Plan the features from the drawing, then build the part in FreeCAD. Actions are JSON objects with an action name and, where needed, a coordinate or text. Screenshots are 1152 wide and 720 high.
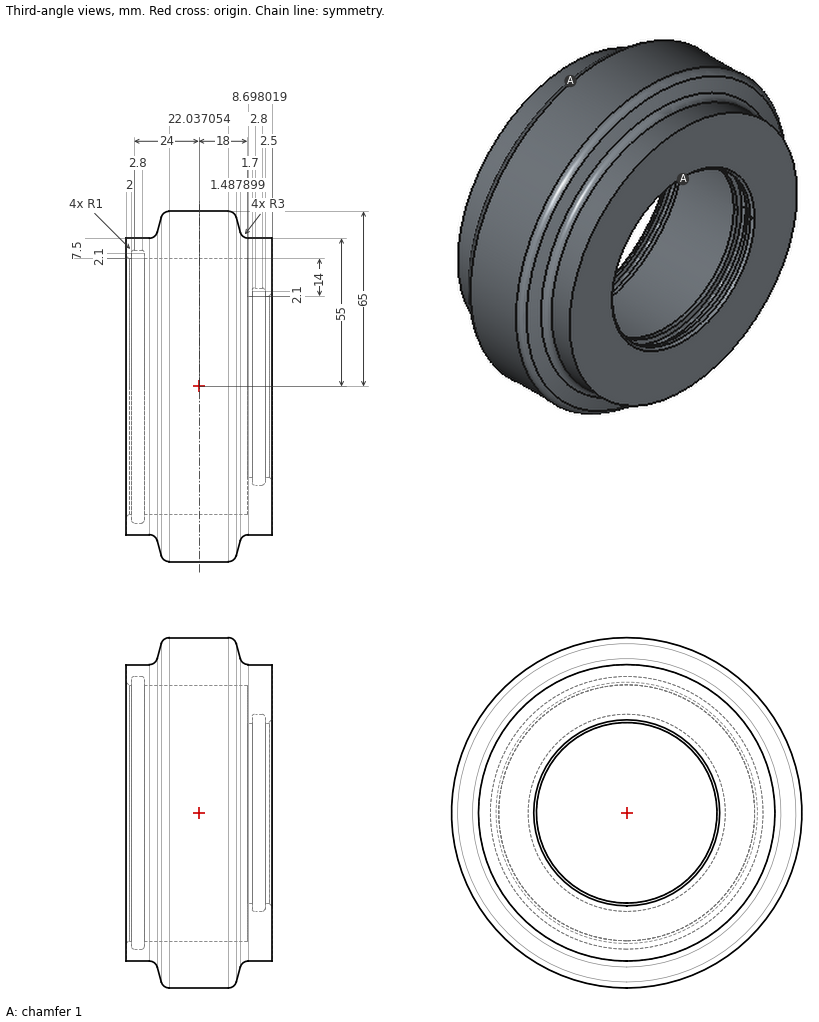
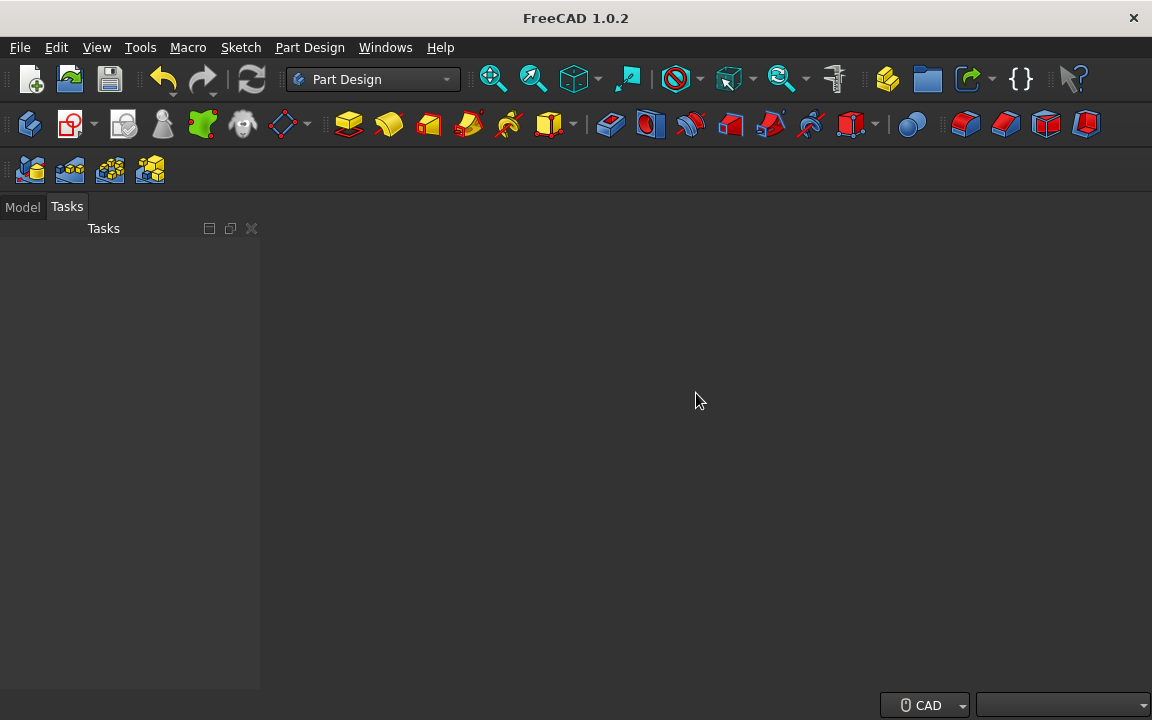
{"action": "key", "text": "ctrl+n"}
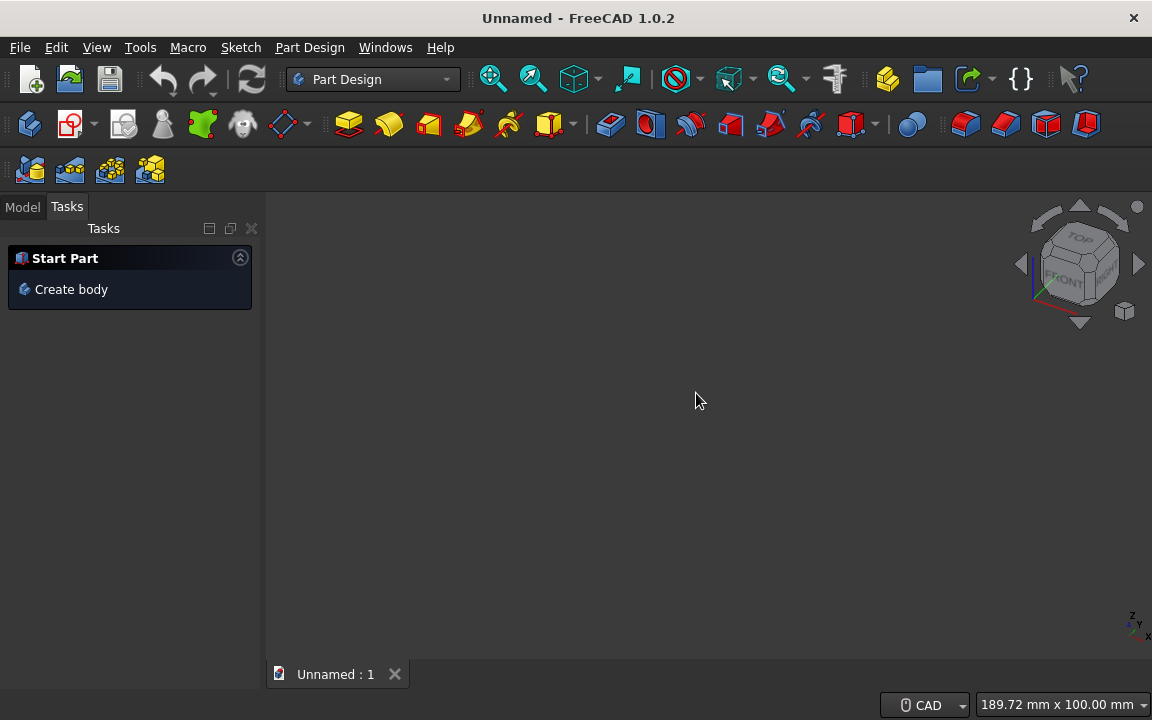
{"action": "left_click", "coordinate": [70, 124]}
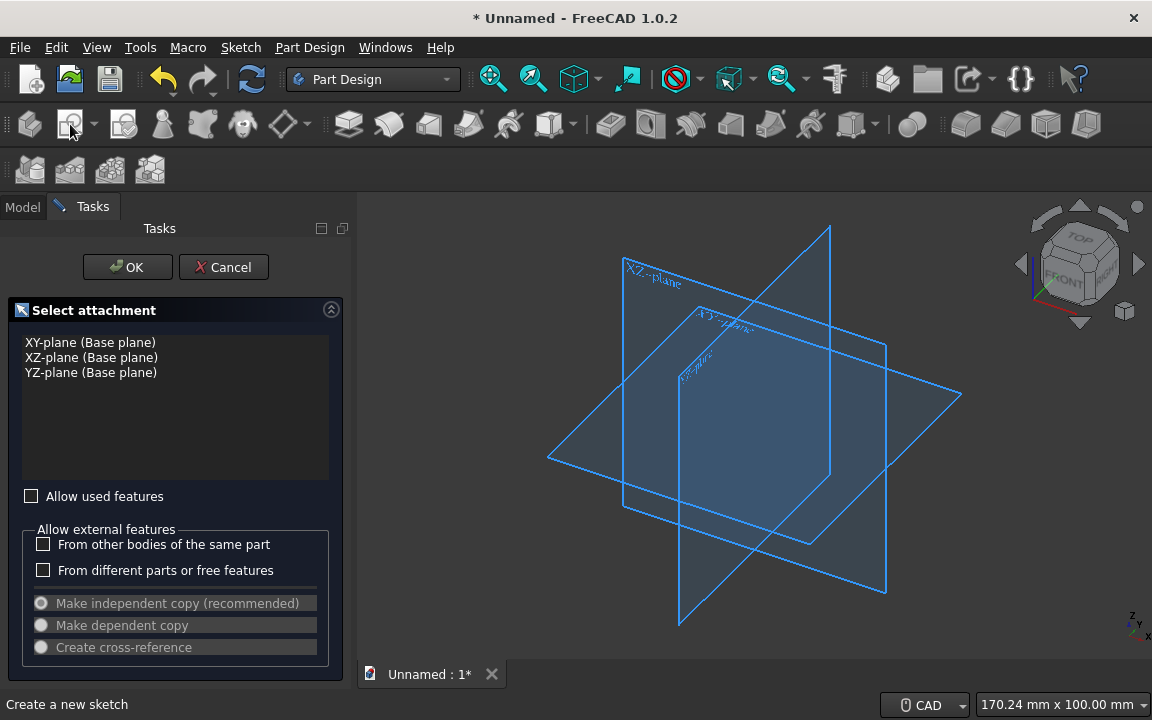
{"action": "left_click", "coordinate": [82, 342]}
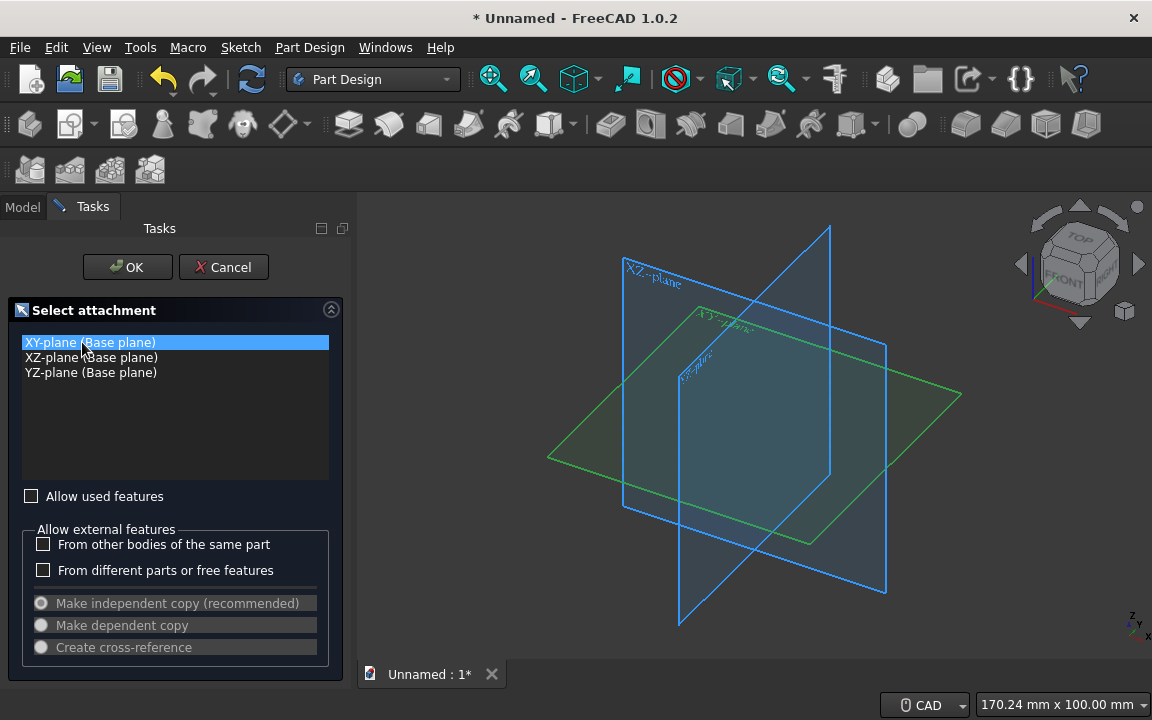
{"action": "left_click", "coordinate": [128, 267]}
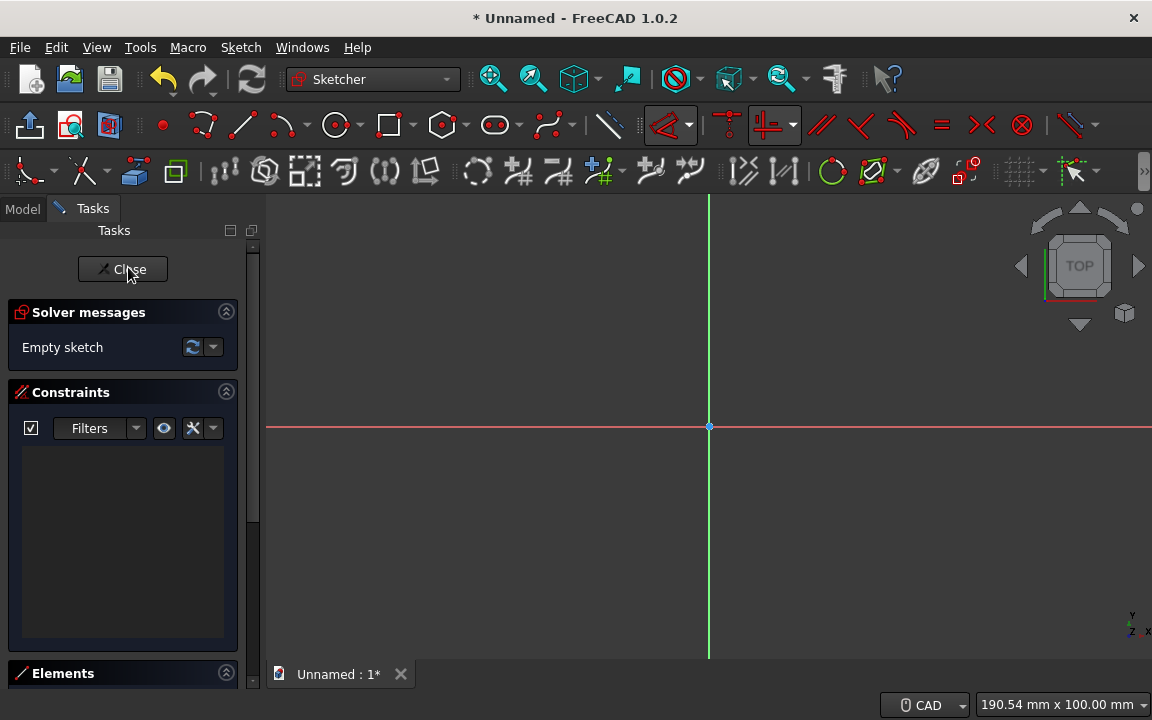
{"action": "scroll", "coordinate": [501, 631], "scroll_direction": "down", "scroll_amount": 2}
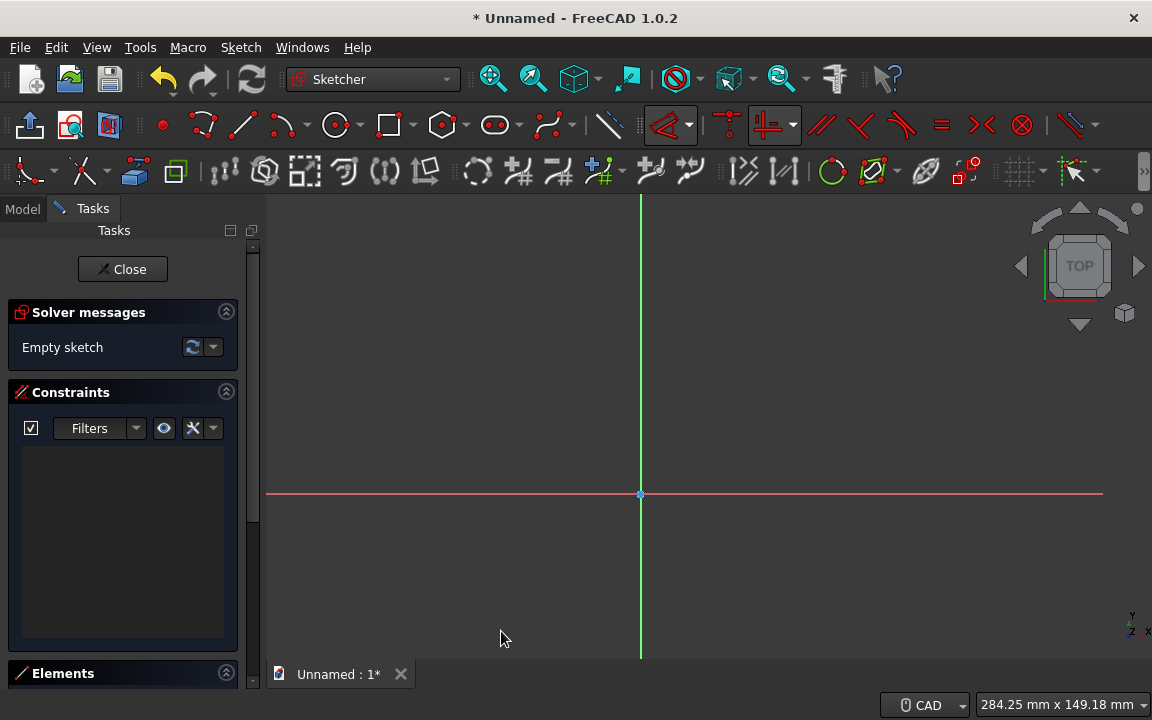
{"action": "scroll", "coordinate": [641, 325], "scroll_direction": "up", "scroll_amount": 2}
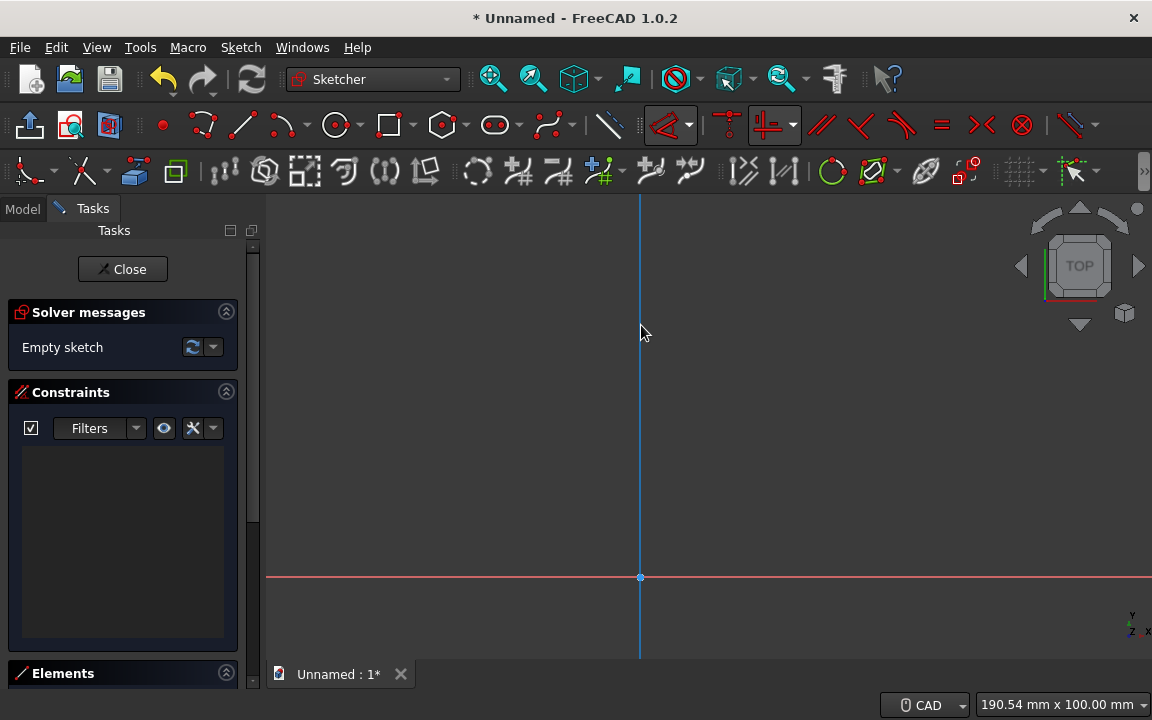
{"action": "key", "text": "g l"}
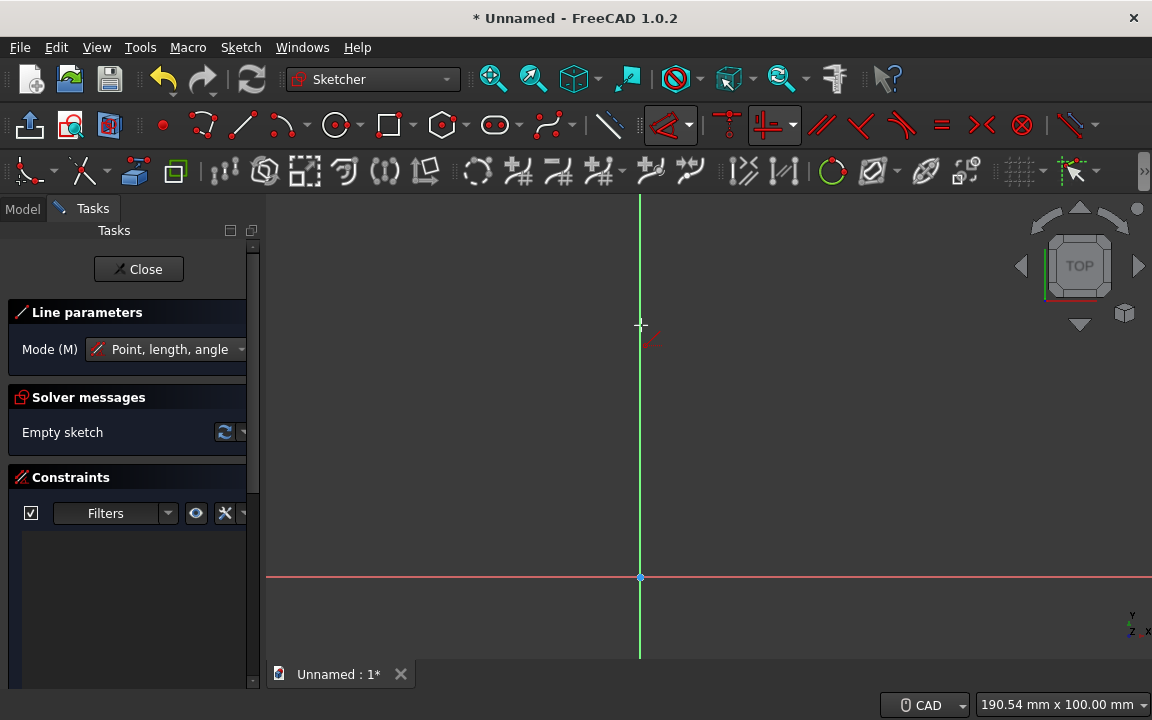
{"action": "left_click", "coordinate": [528, 342]}
{"action": "left_click", "coordinate": [541, 342]}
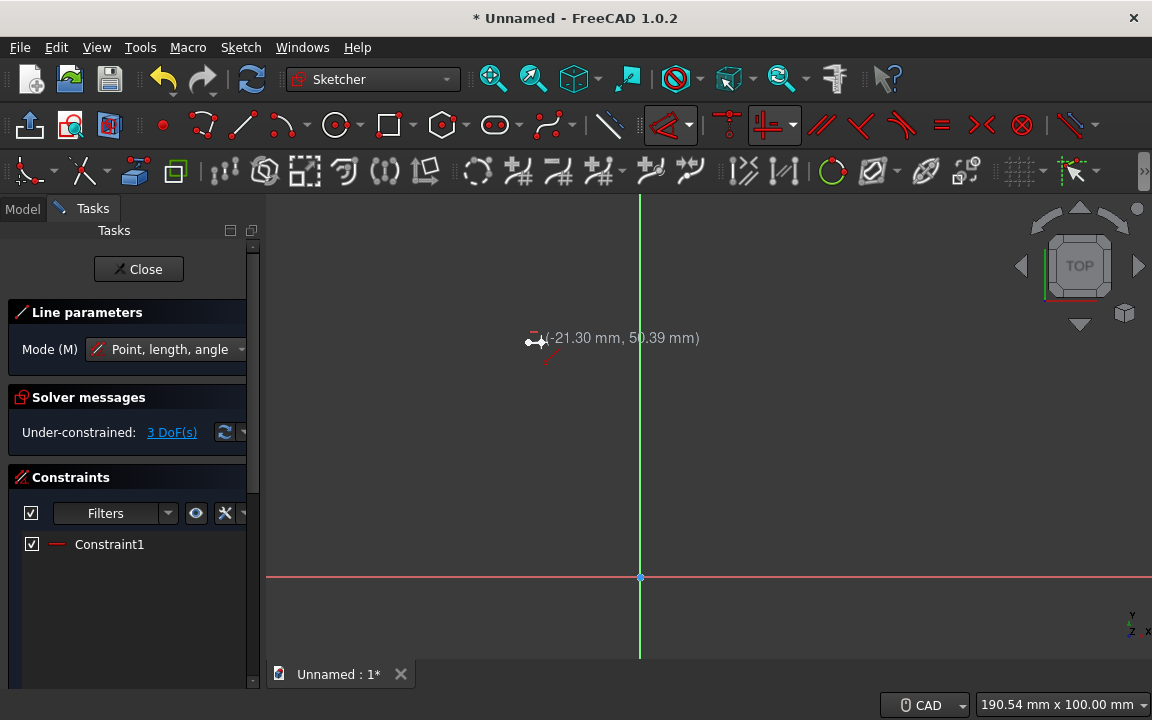
{"action": "key", "text": "g m"}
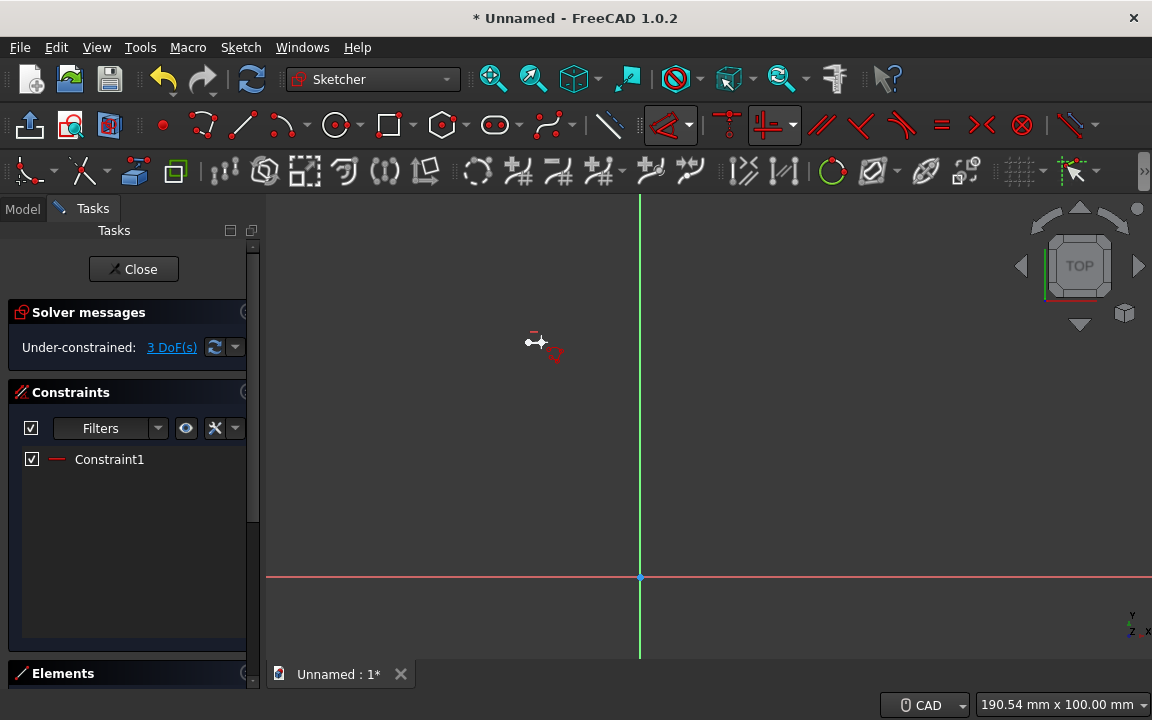
{"action": "scroll", "coordinate": [546, 347], "scroll_direction": "up", "scroll_amount": 5}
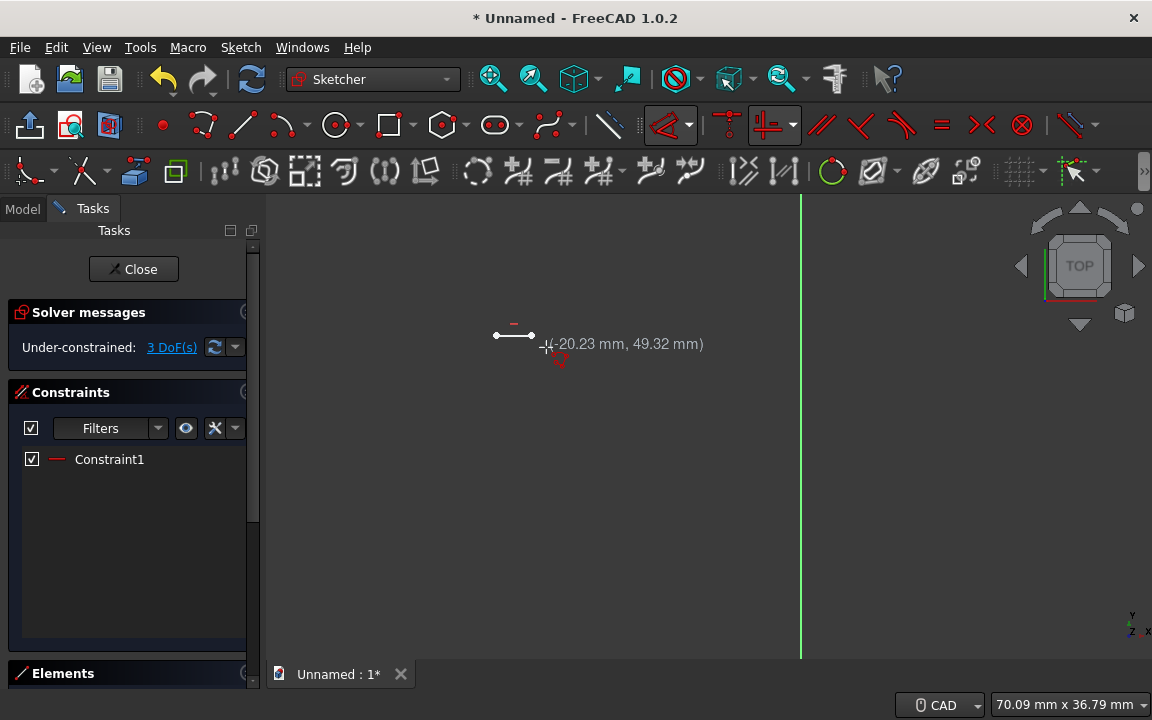
{"action": "left_click", "coordinate": [546, 346]}
{"action": "left_click", "coordinate": [546, 372]}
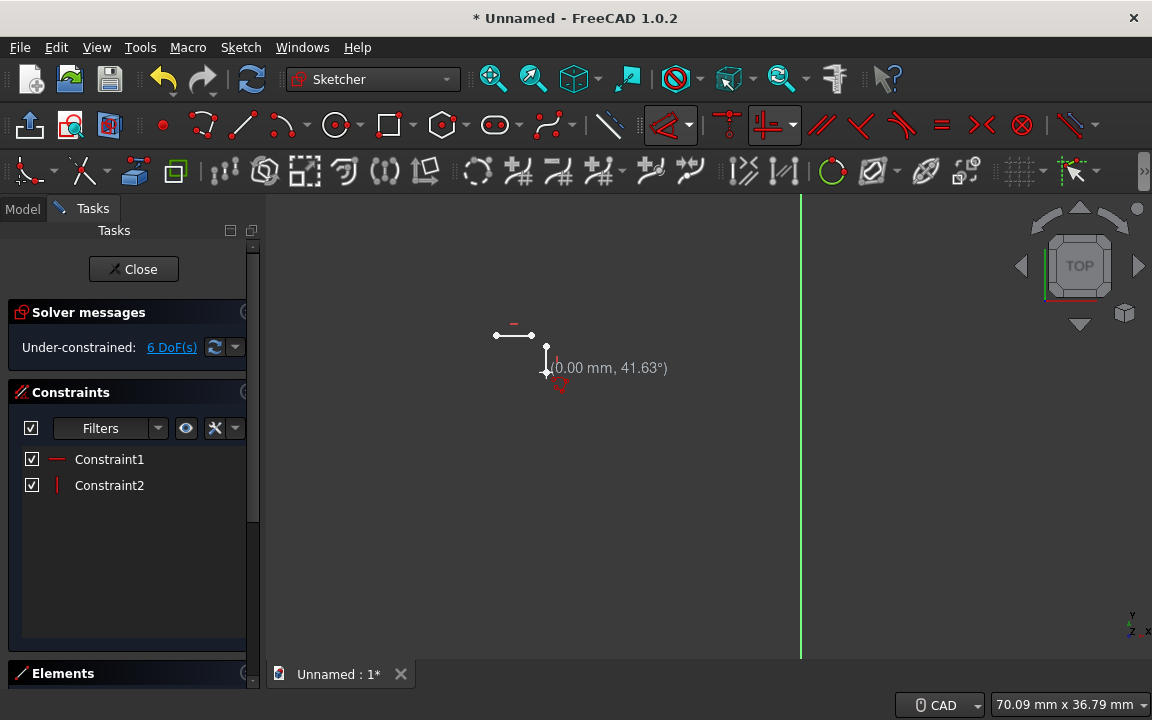
{"action": "scroll", "coordinate": [547, 348], "scroll_direction": "down", "scroll_amount": 5}